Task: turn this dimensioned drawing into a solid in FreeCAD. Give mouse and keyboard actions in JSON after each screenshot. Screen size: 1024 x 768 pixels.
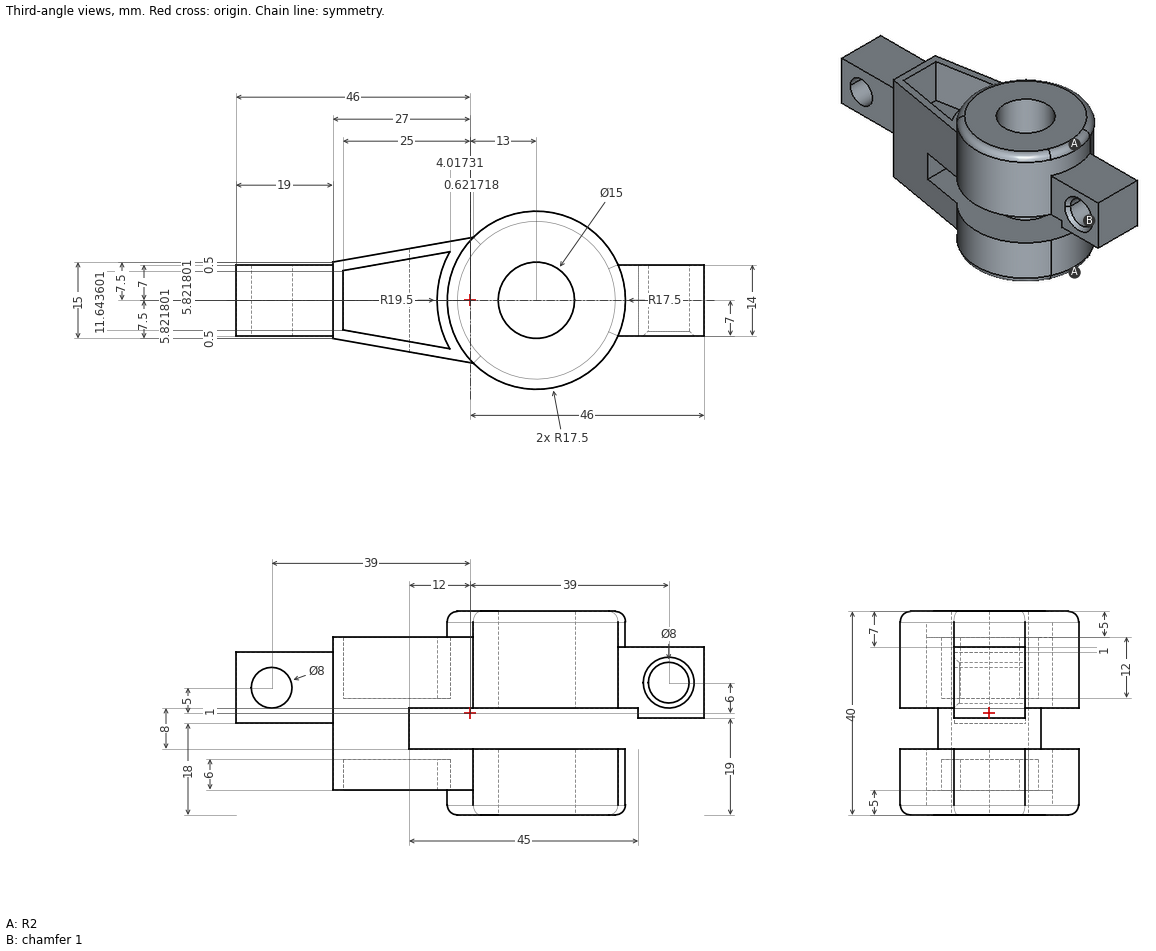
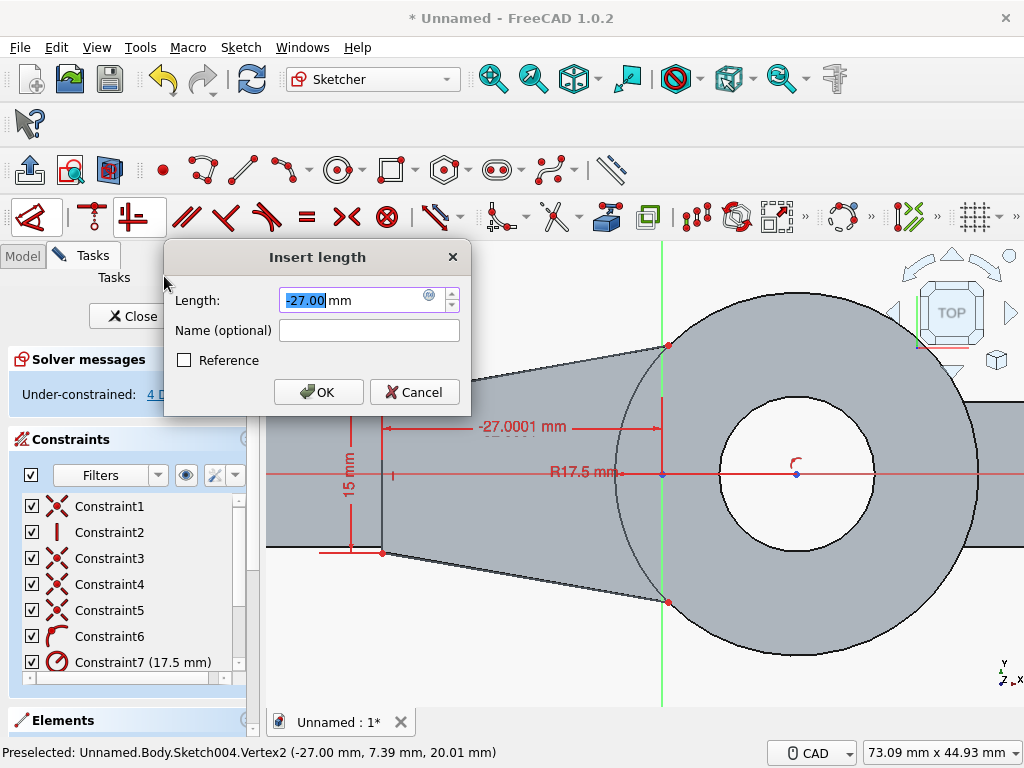
{"action": "type", "text": "-27"}
{"action": "key", "text": "Return"}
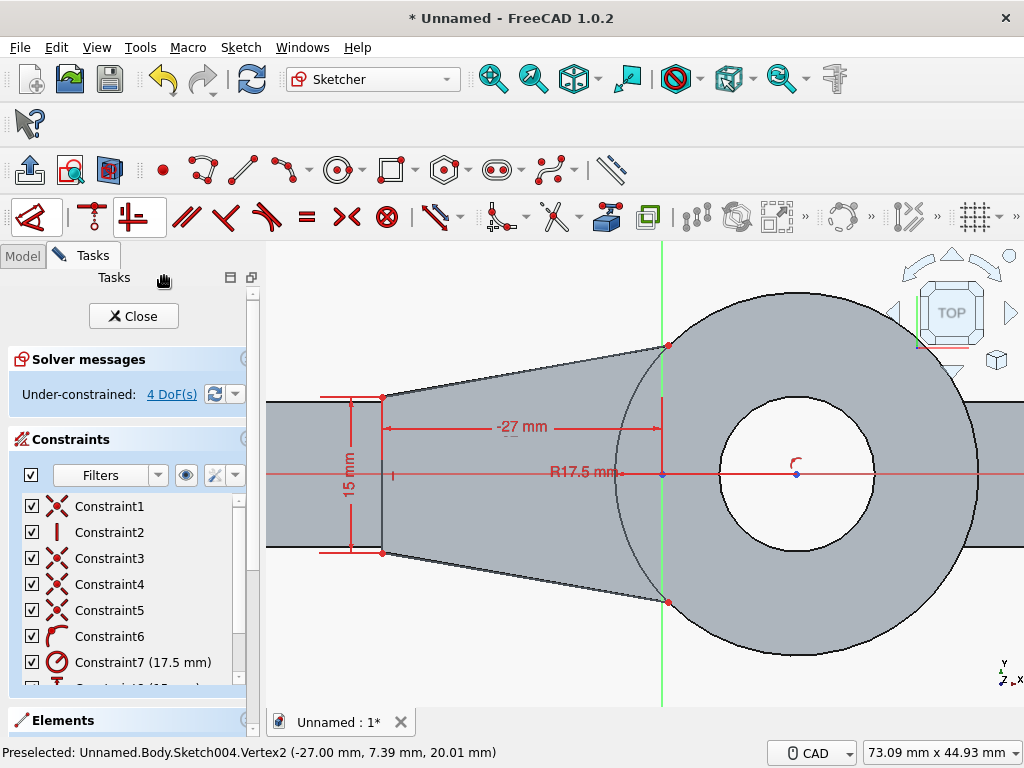
{"action": "left_click", "coordinate": [797, 474]}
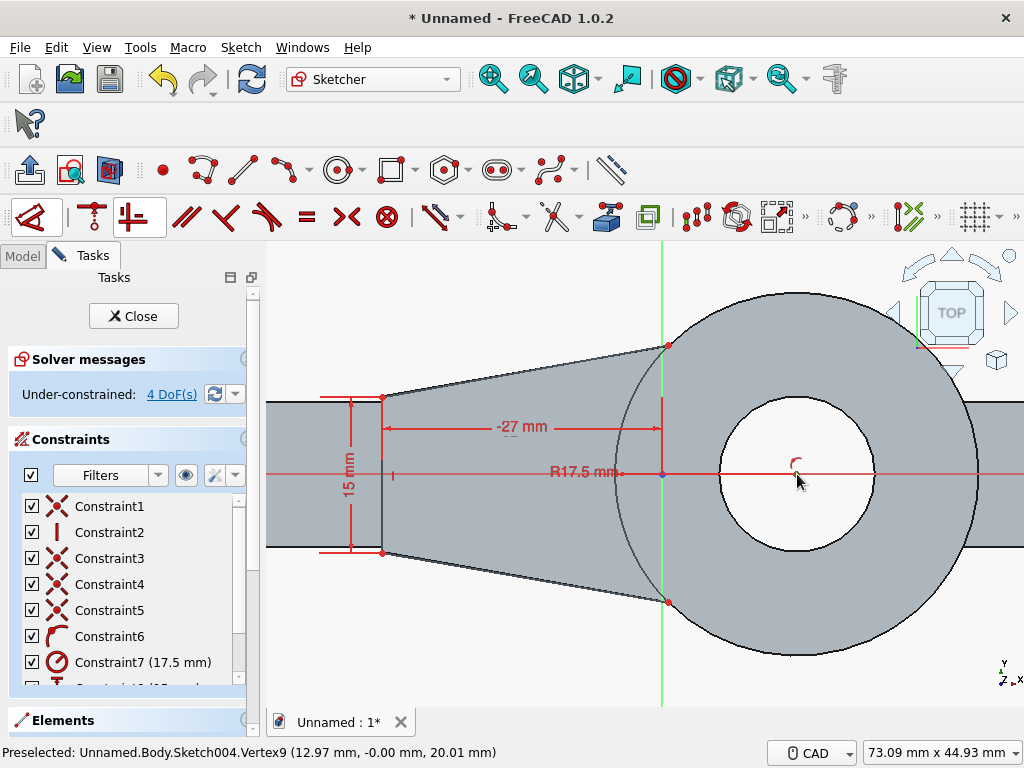
{"action": "key", "text": "l"}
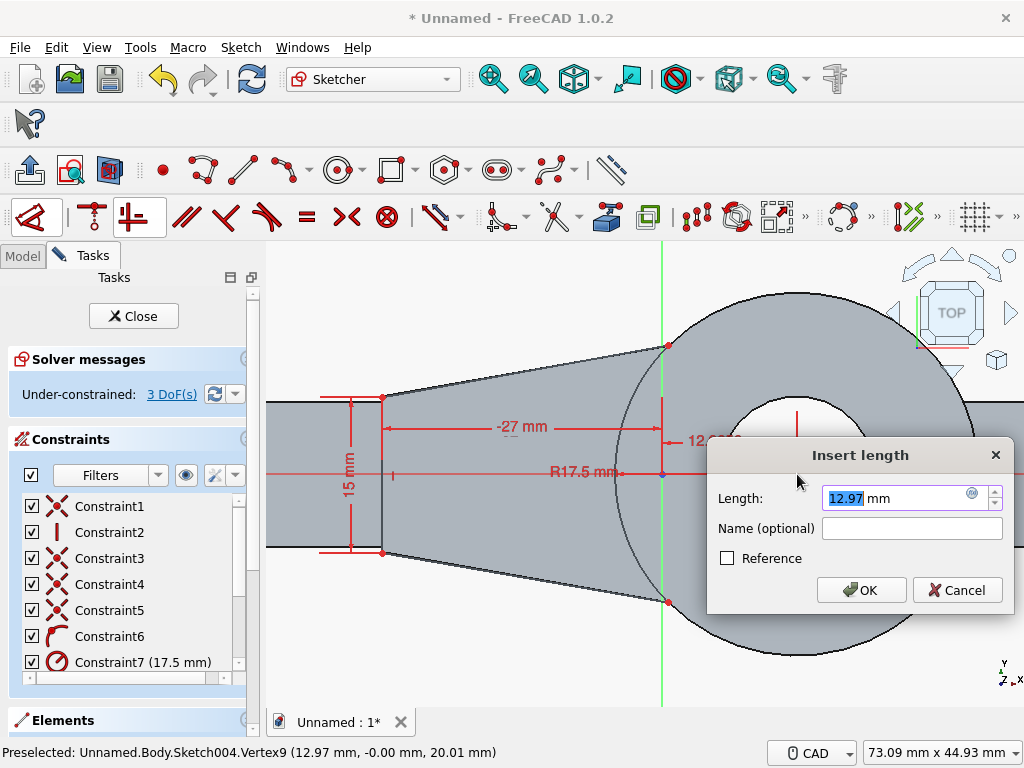
{"action": "type", "text": "13"}
{"action": "key", "text": "Return"}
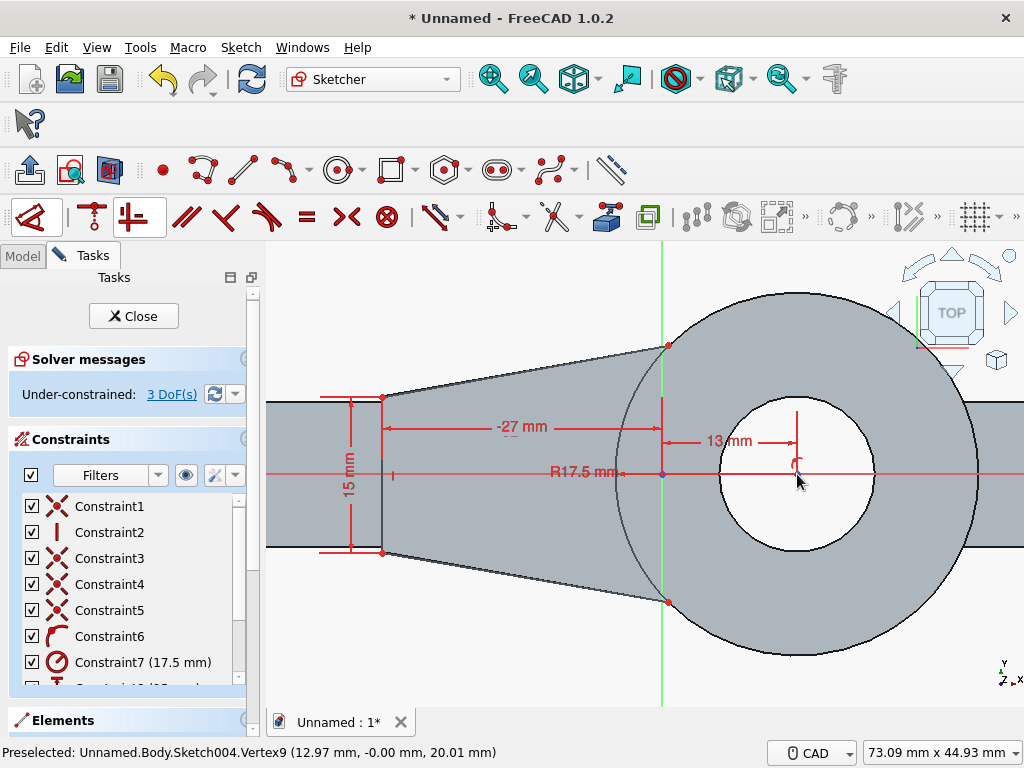
{"action": "left_click", "coordinate": [382, 397]}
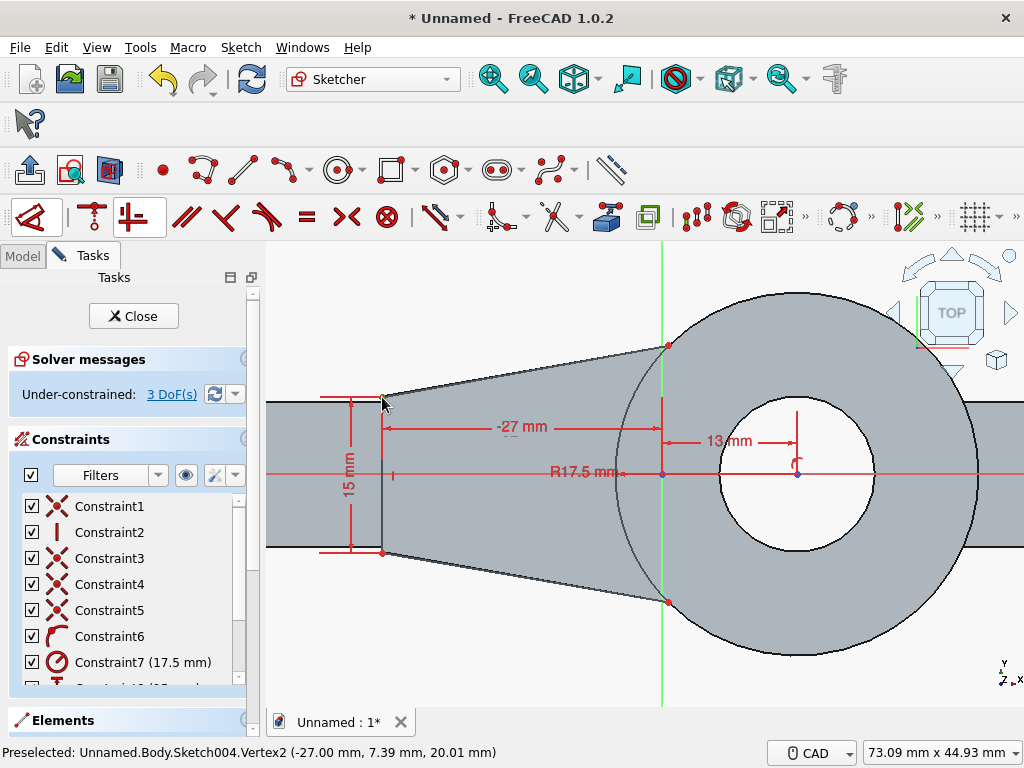
{"action": "left_click", "coordinate": [56, 218]}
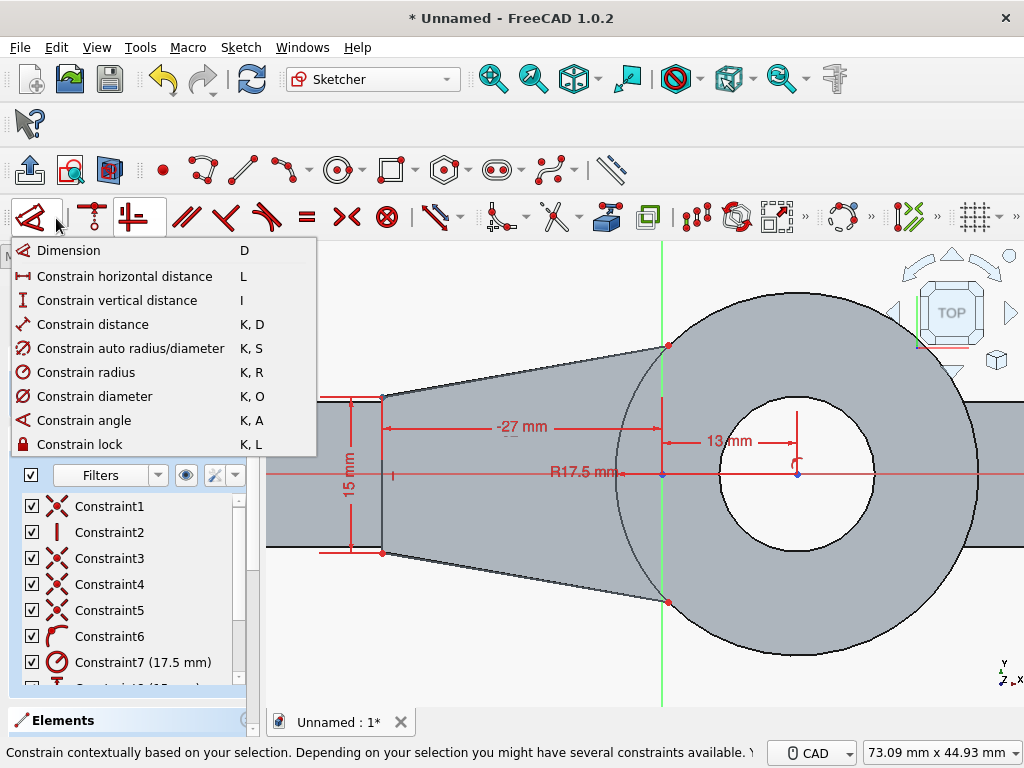
{"action": "left_click", "coordinate": [164, 300]}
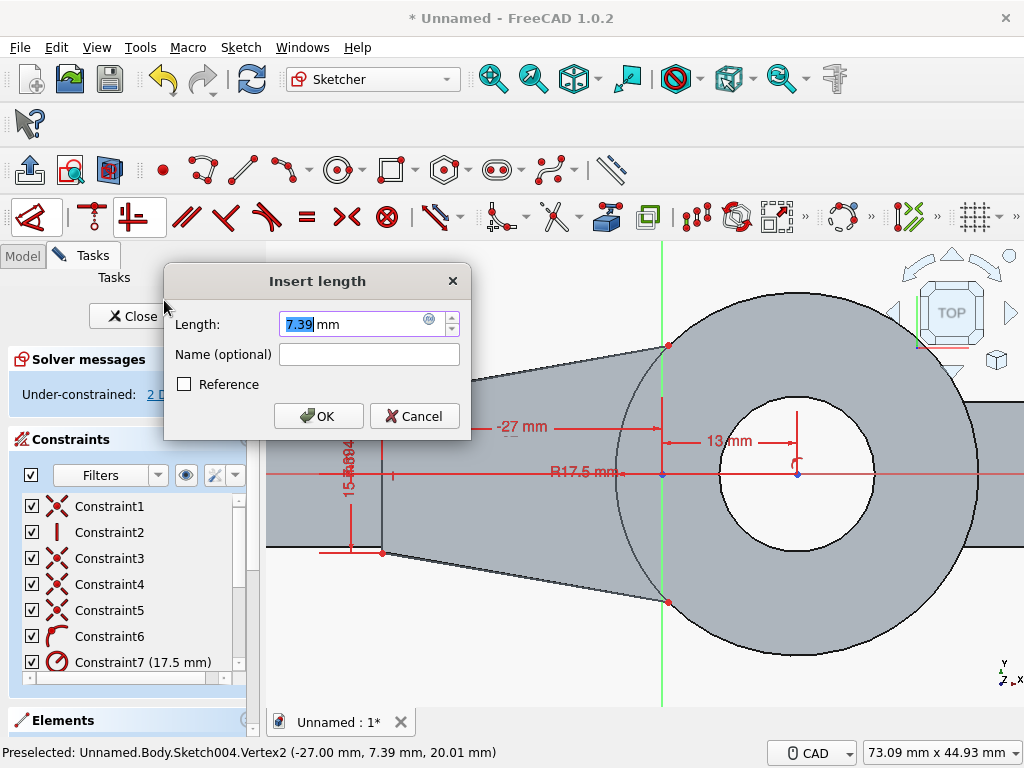
{"action": "type", "text": "7.5"}
{"action": "key", "text": "Return"}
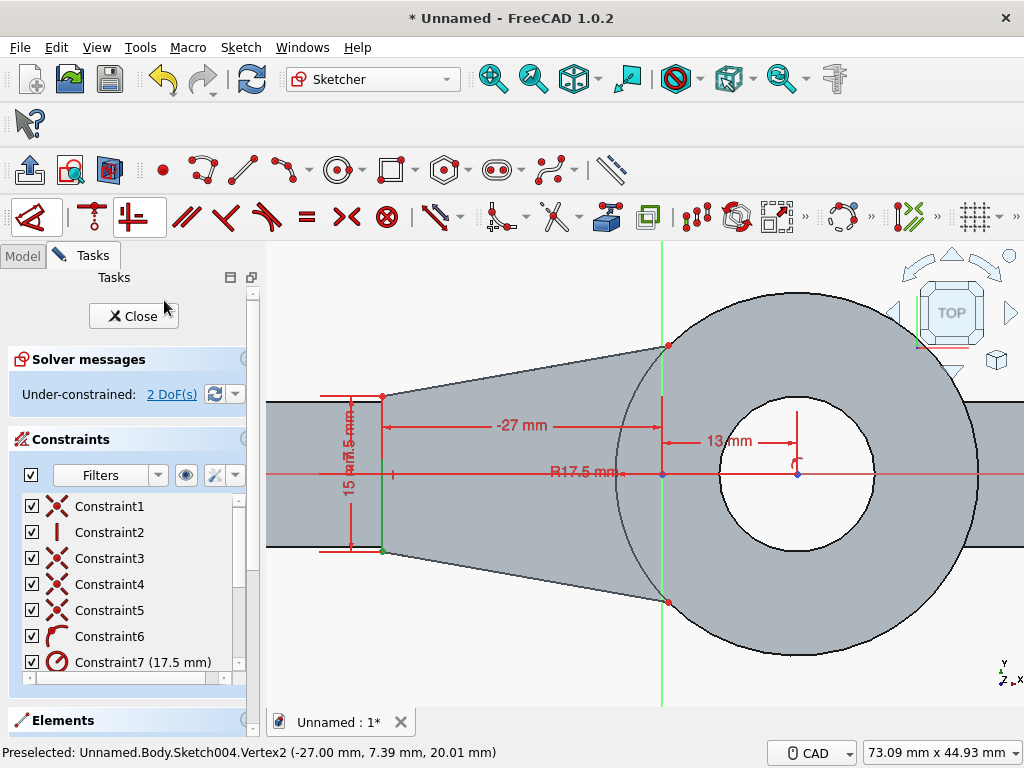
{"action": "scroll", "coordinate": [669, 346], "scroll_direction": "up", "scroll_amount": 10}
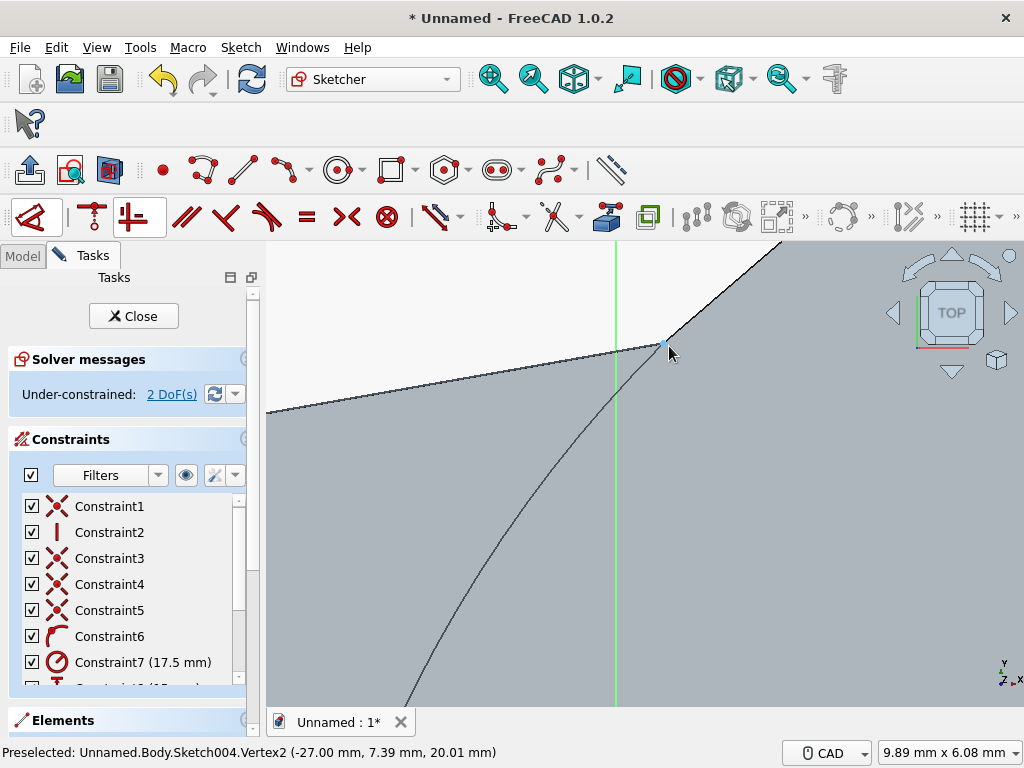
{"action": "left_click", "coordinate": [664, 343]}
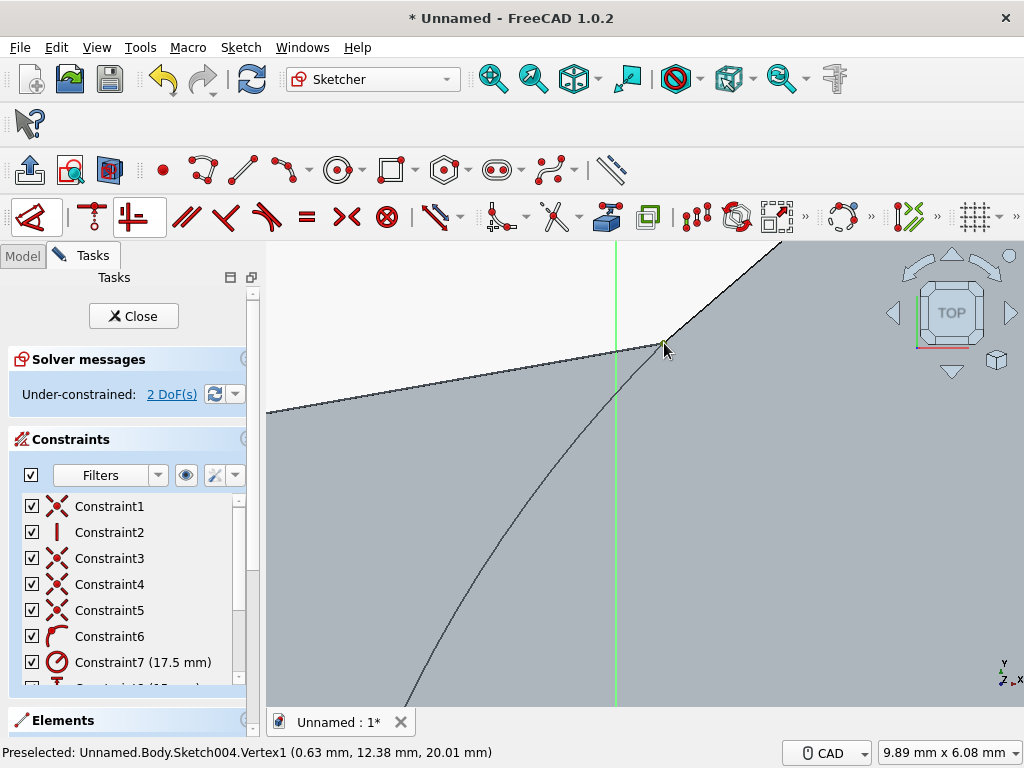
{"action": "key", "text": "l"}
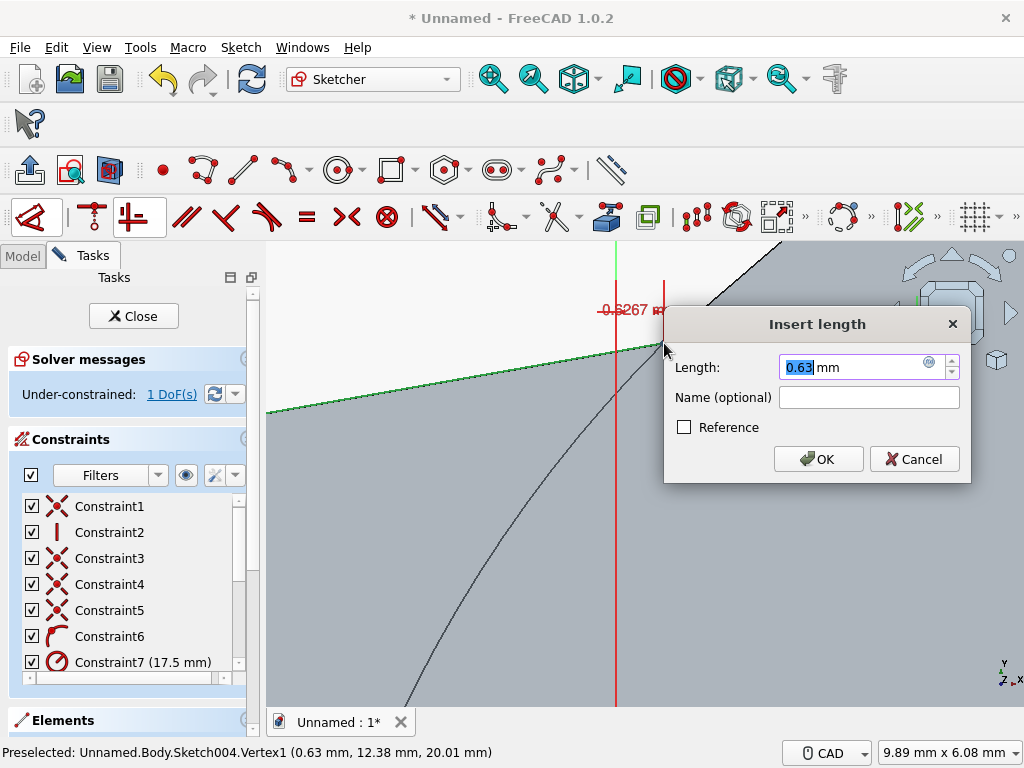
{"action": "type", "text": "0.621718"}
{"action": "key", "text": "Return"}